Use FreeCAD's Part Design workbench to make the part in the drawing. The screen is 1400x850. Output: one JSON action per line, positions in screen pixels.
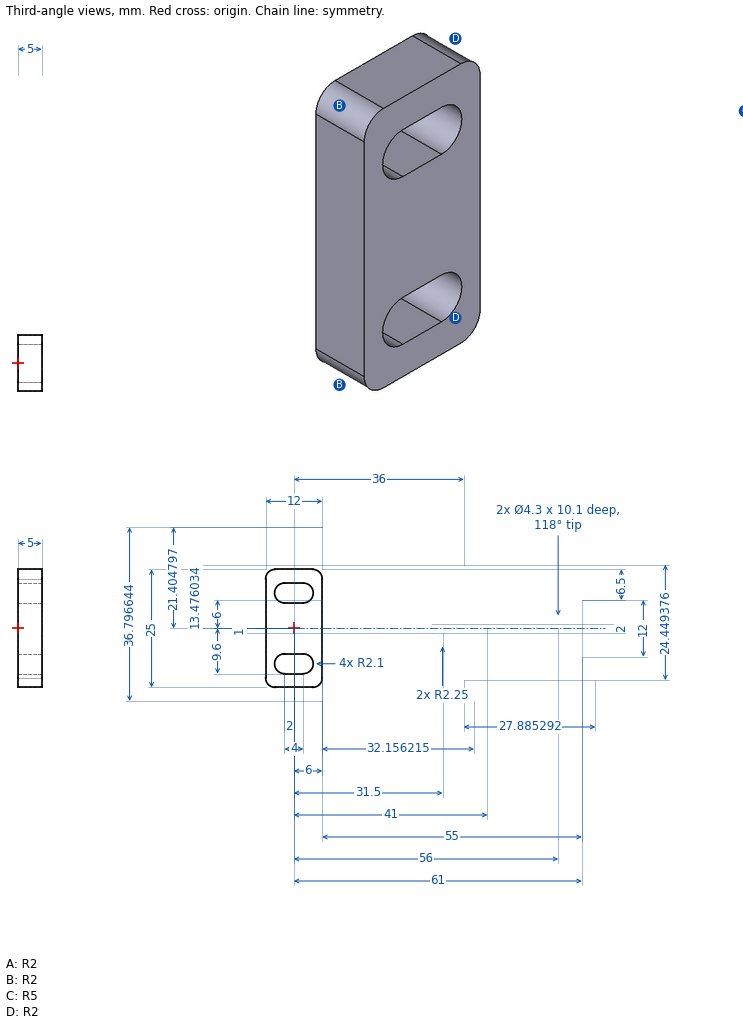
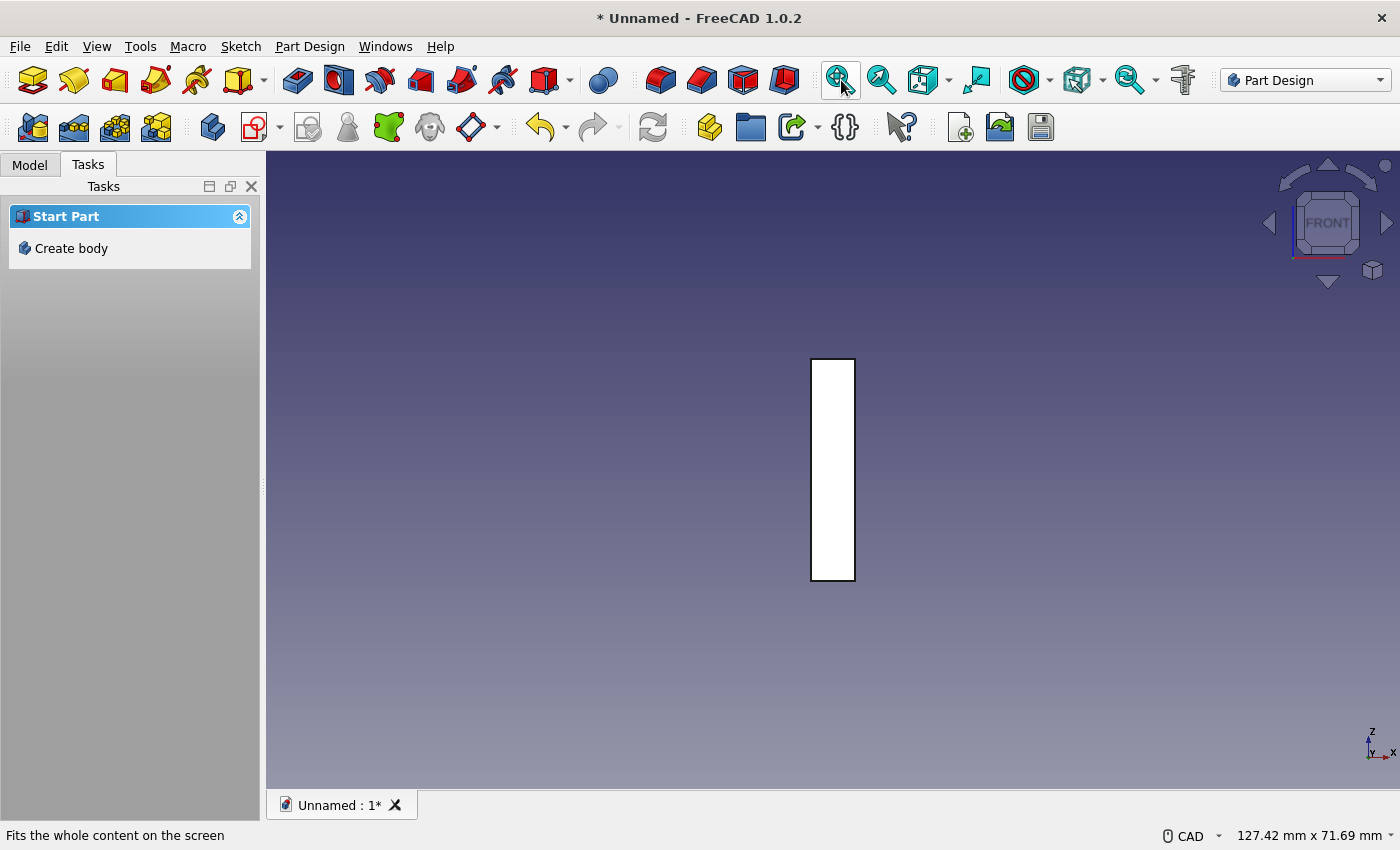
{"action": "key", "text": "5"}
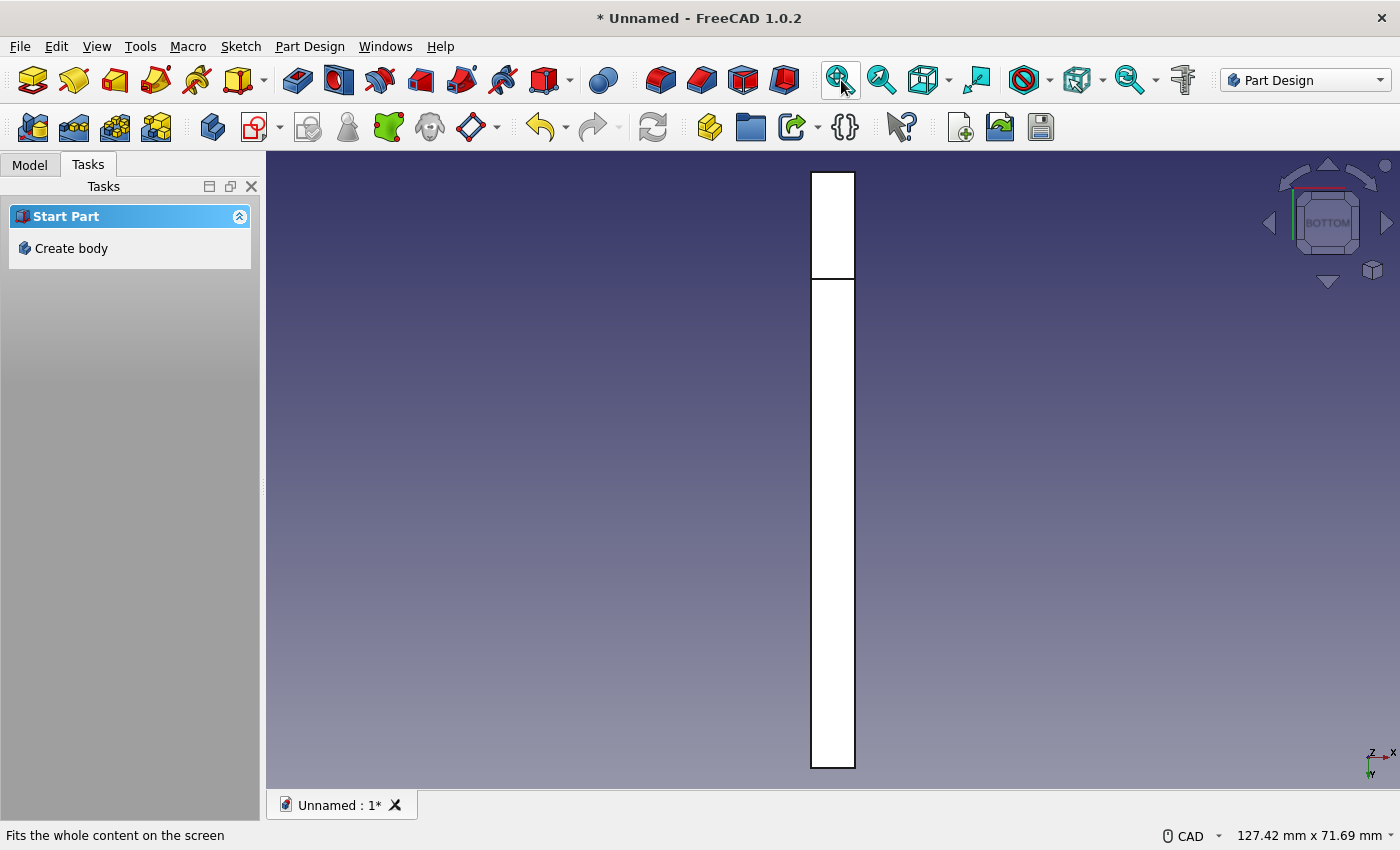
{"action": "key", "text": "4"}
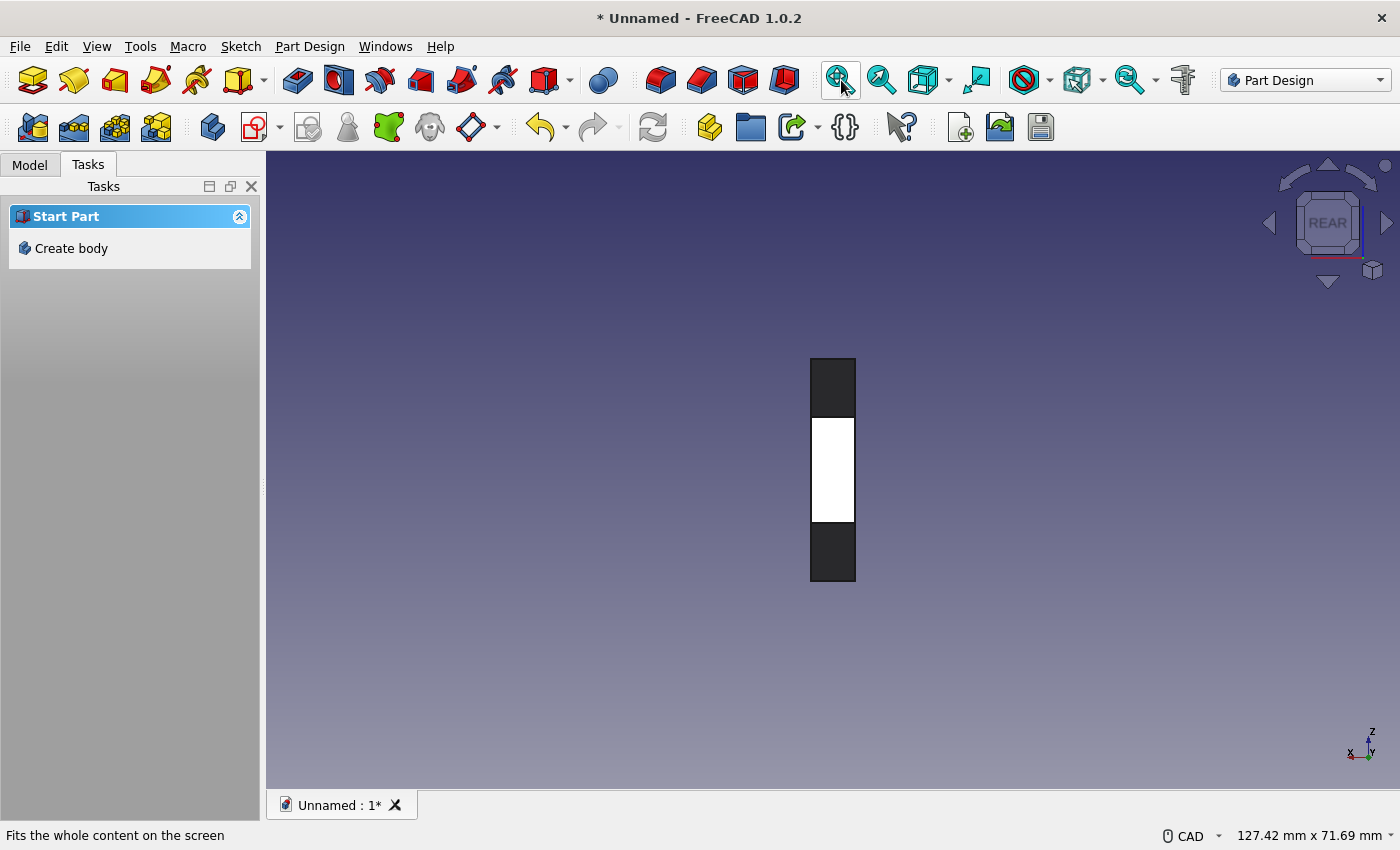
{"action": "left_click", "coordinate": [841, 80]}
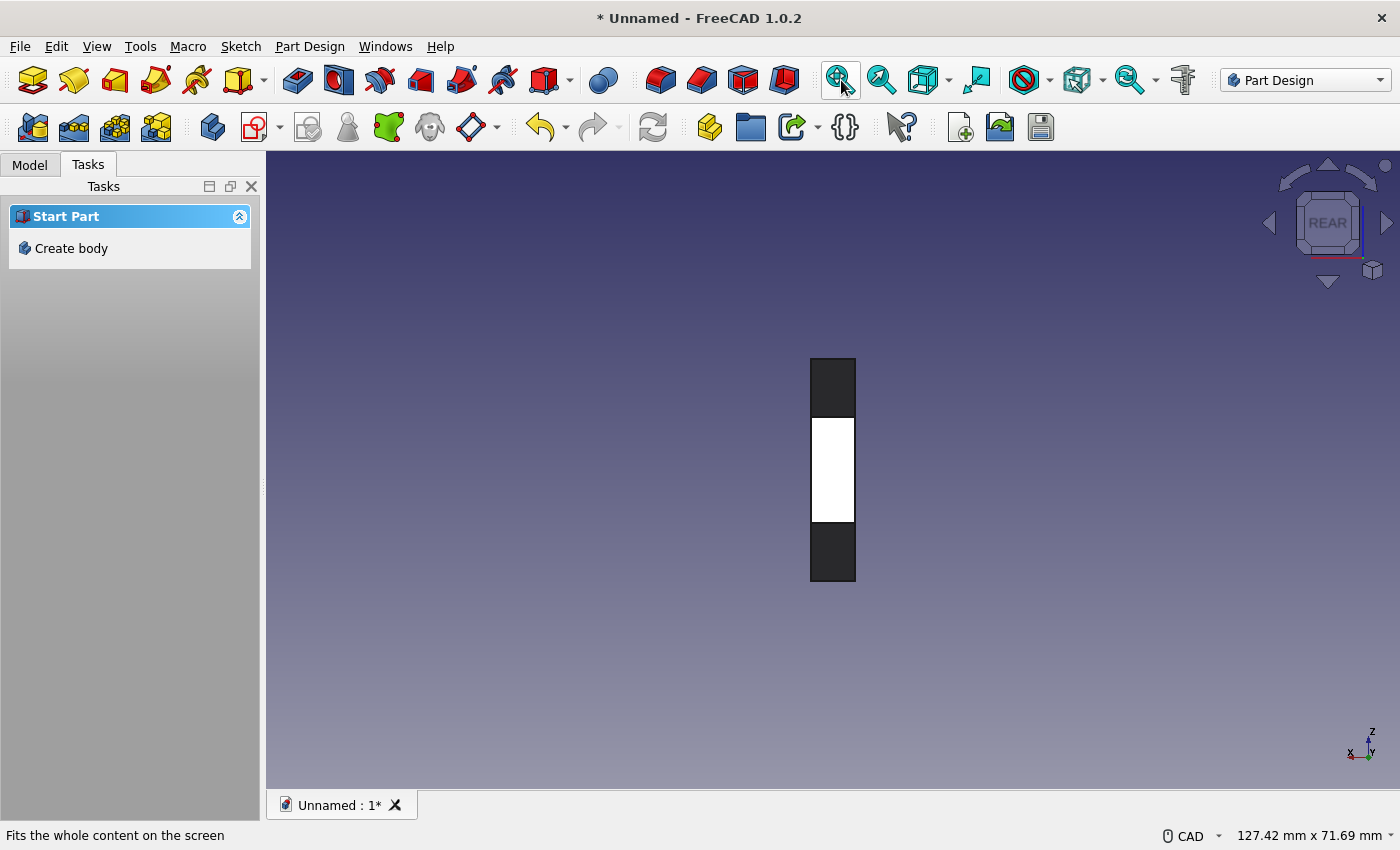
{"action": "left_click", "coordinate": [833, 416]}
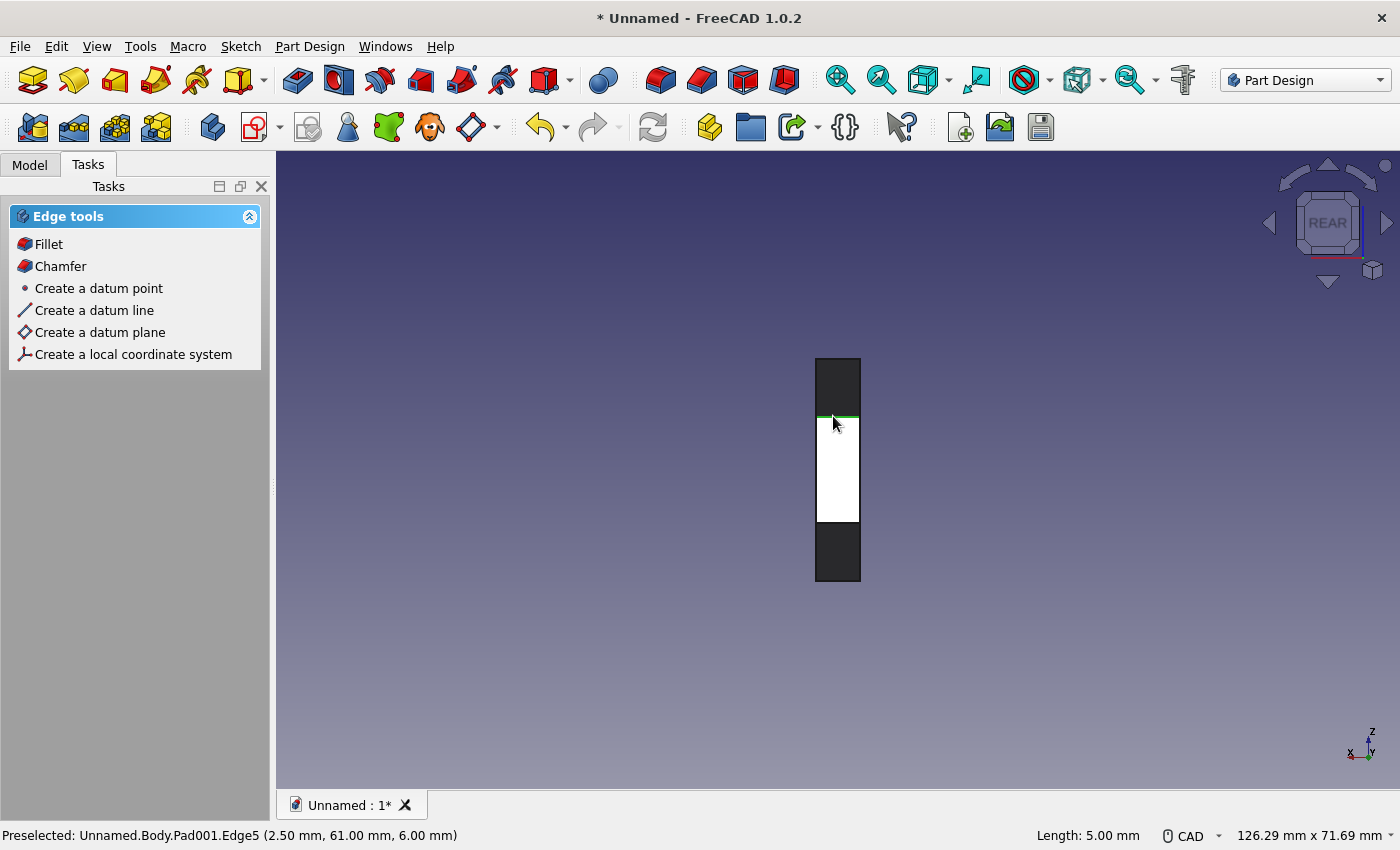
{"action": "left_click", "coordinate": [838, 522], "text": "ctrl"}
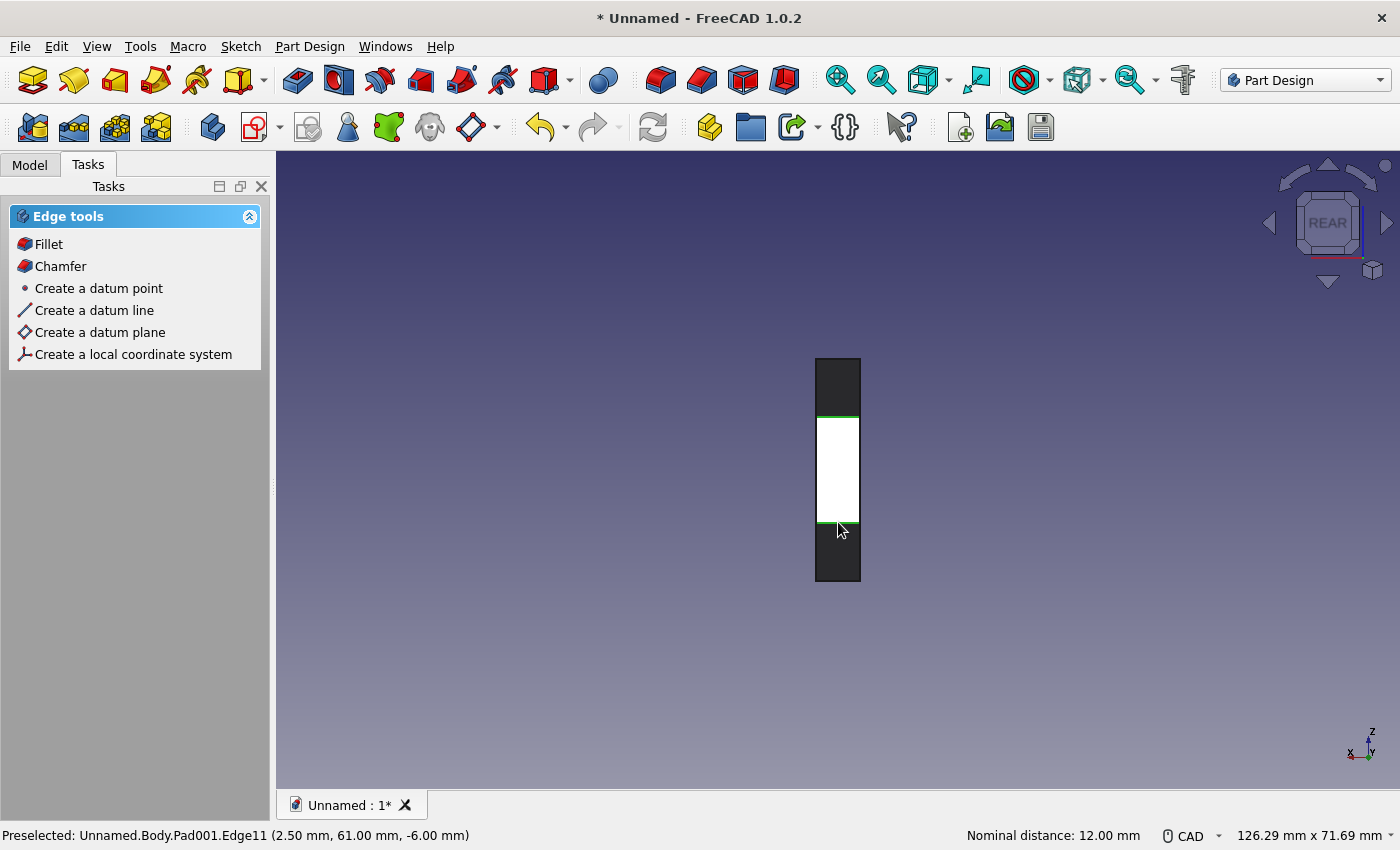
{"action": "left_click", "coordinate": [661, 80]}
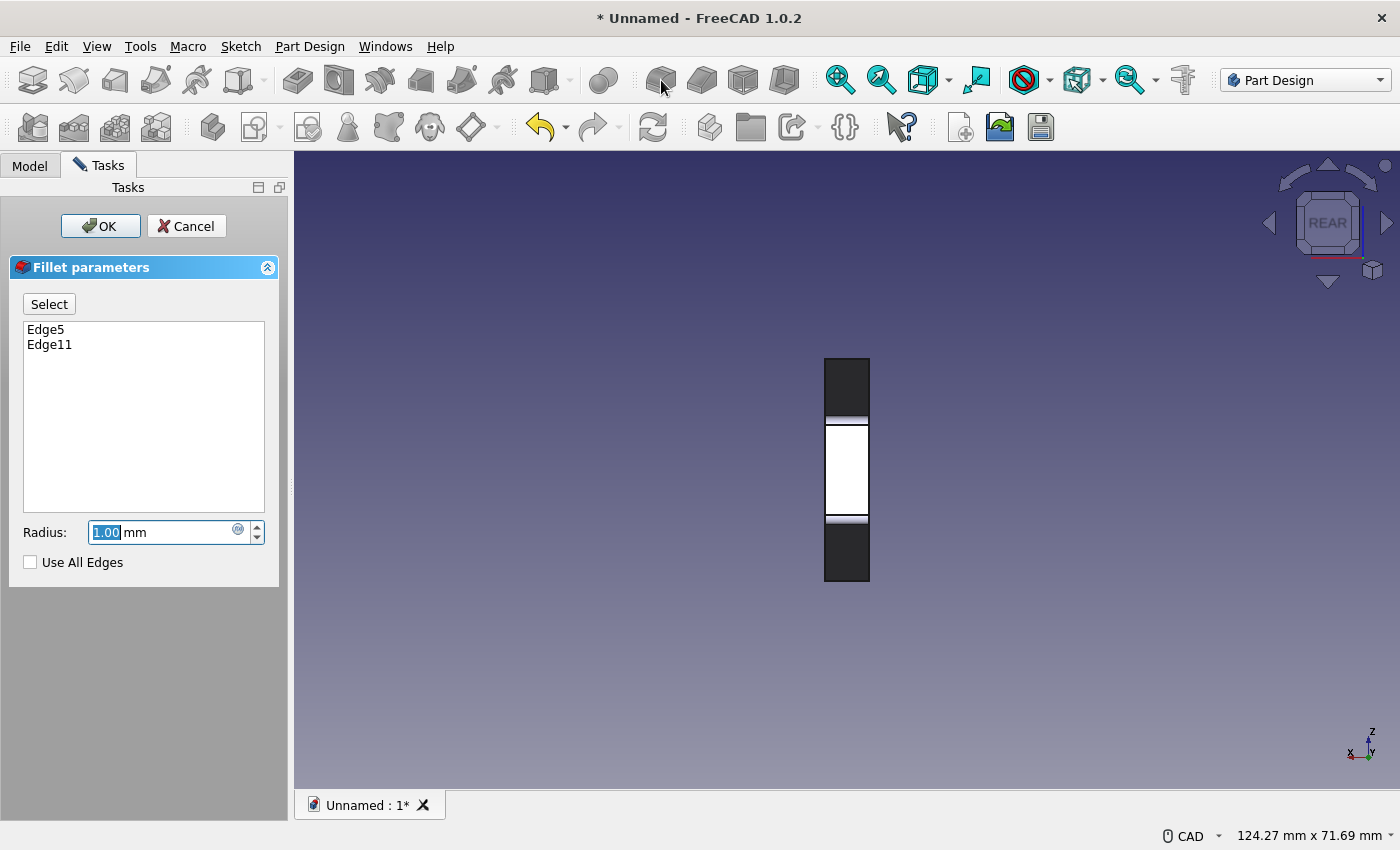
{"action": "type", "text": "2"}
{"action": "key", "text": "Tab"}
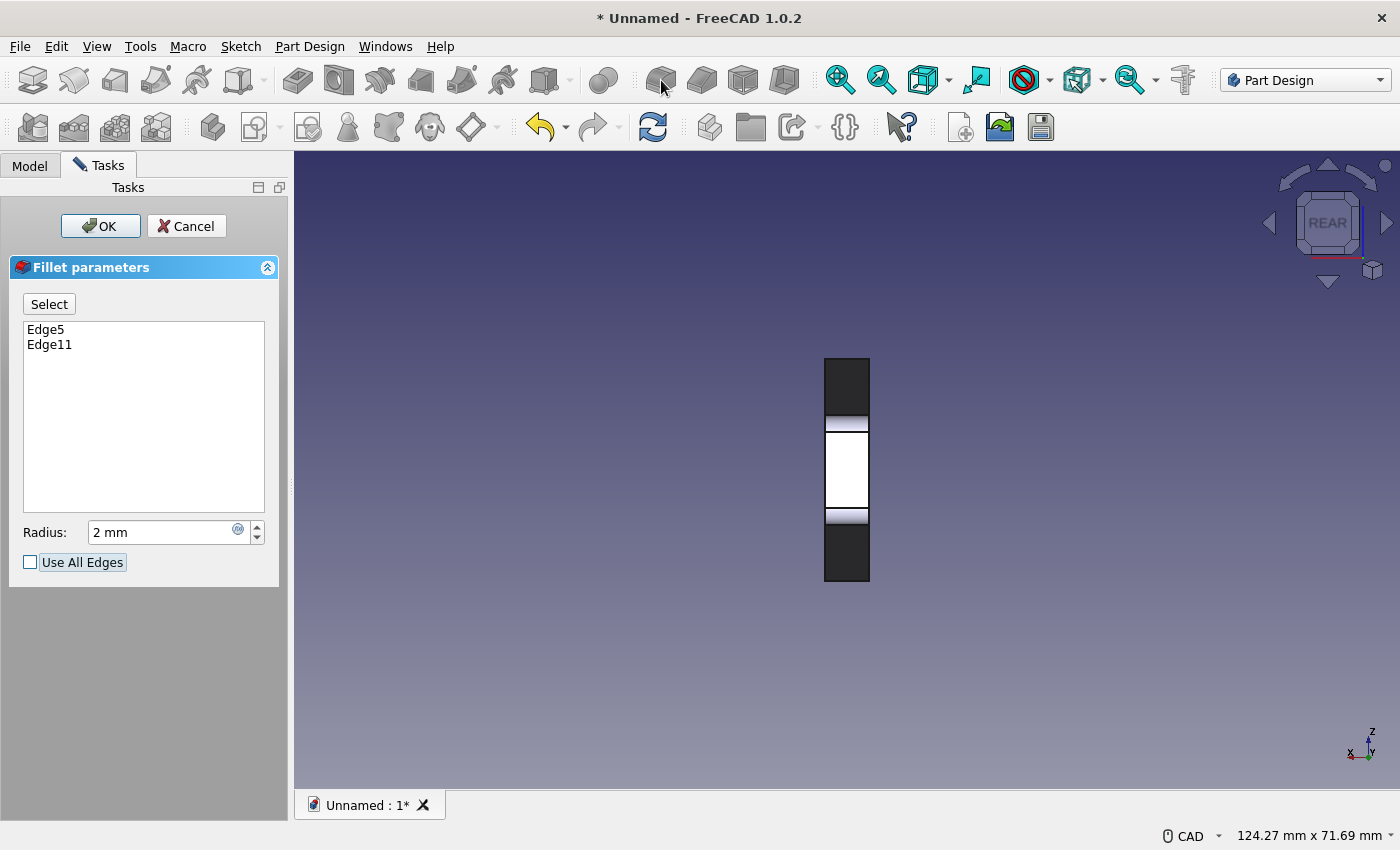
{"action": "left_click", "coordinate": [101, 226]}